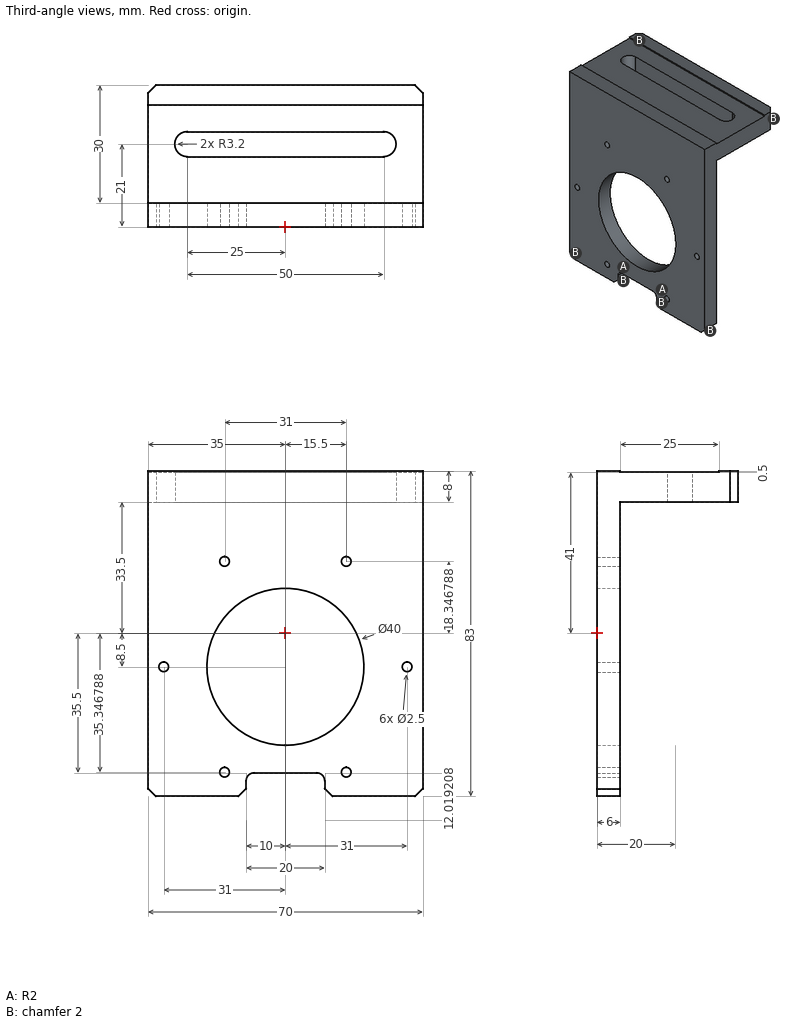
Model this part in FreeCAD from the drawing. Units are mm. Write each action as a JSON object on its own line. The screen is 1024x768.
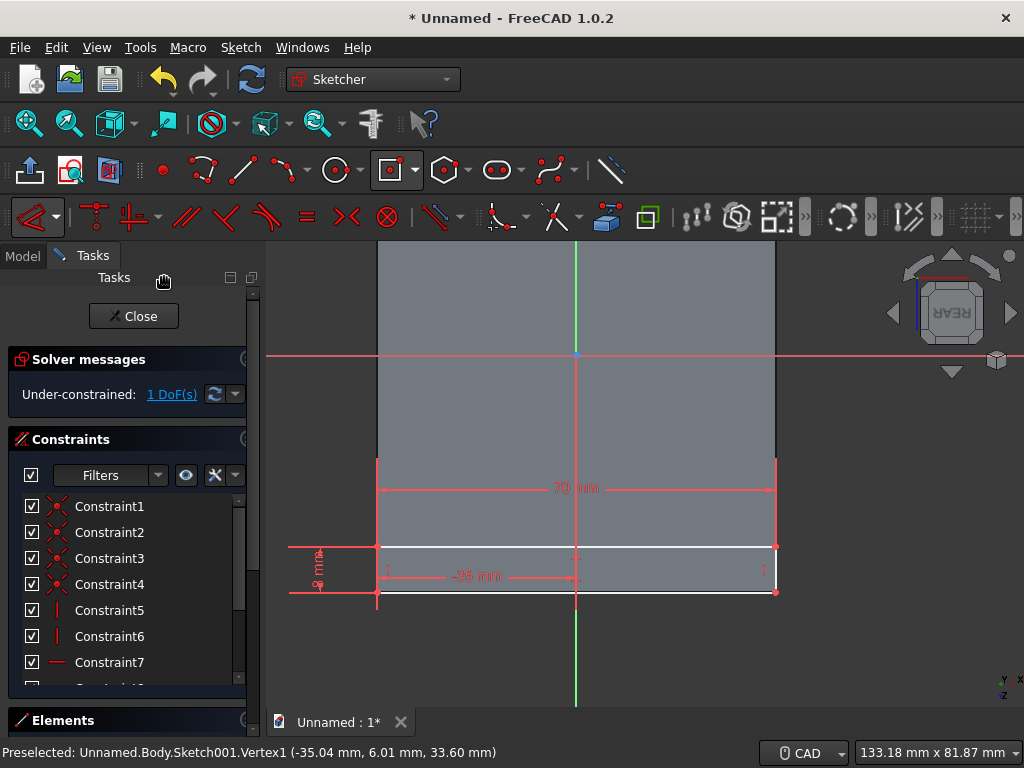
{"action": "left_click", "coordinate": [377, 547]}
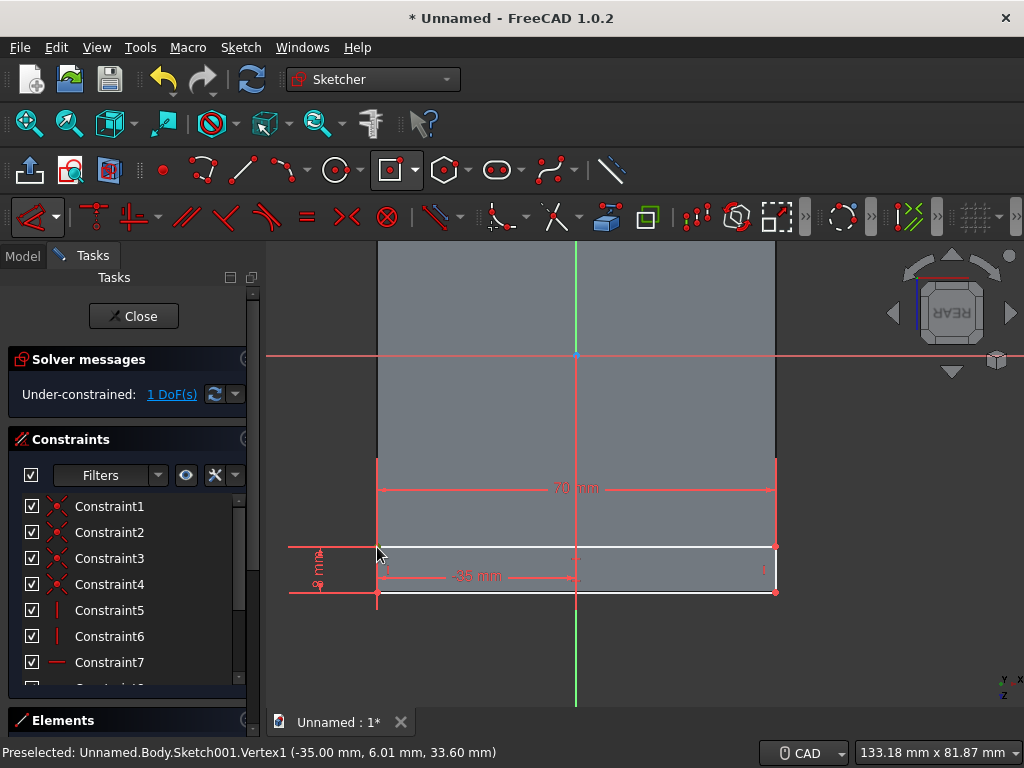
{"action": "left_click", "coordinate": [58, 218]}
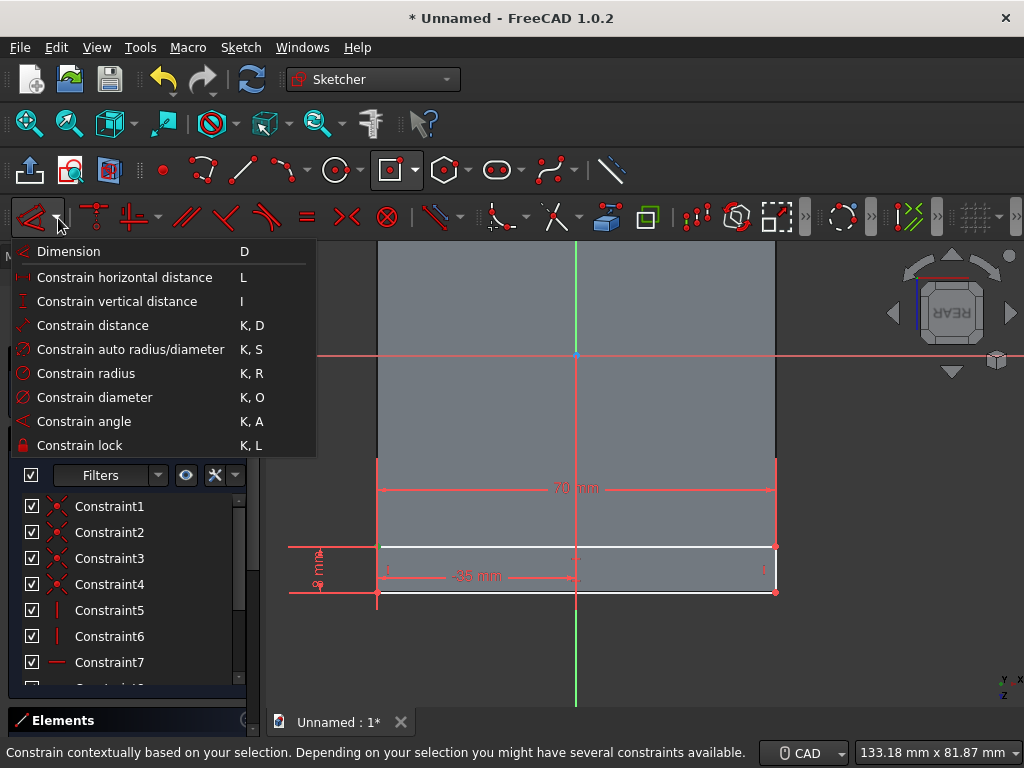
{"action": "left_click", "coordinate": [164, 301]}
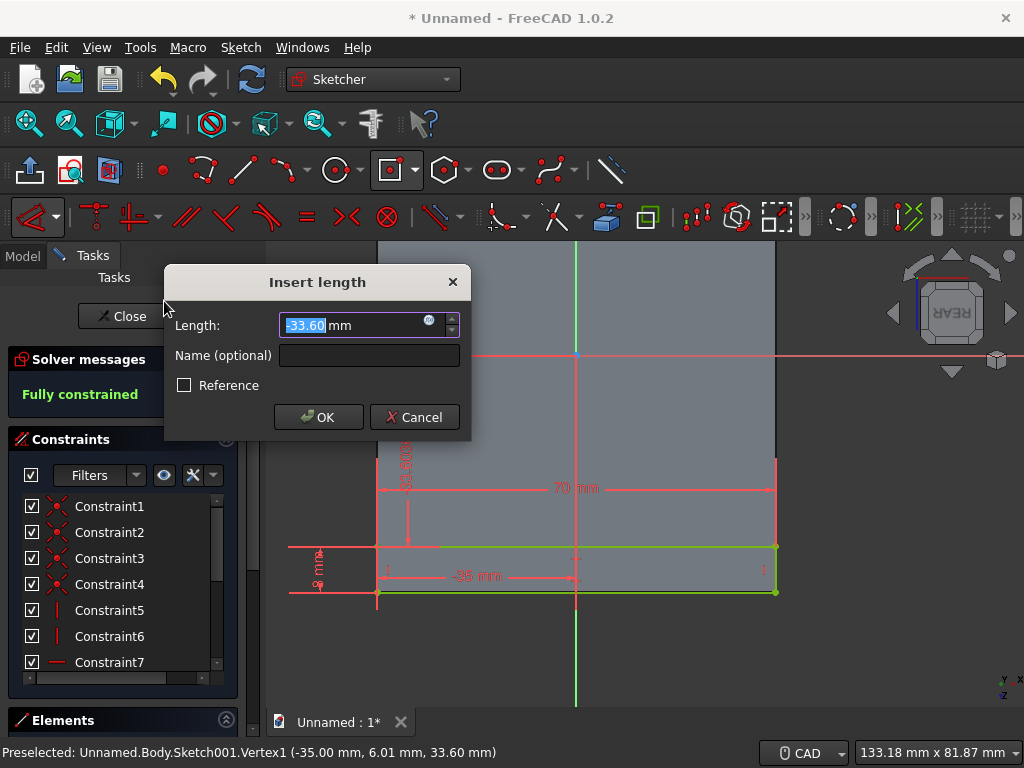
{"action": "type", "text": "-33.5"}
{"action": "key", "text": "Return"}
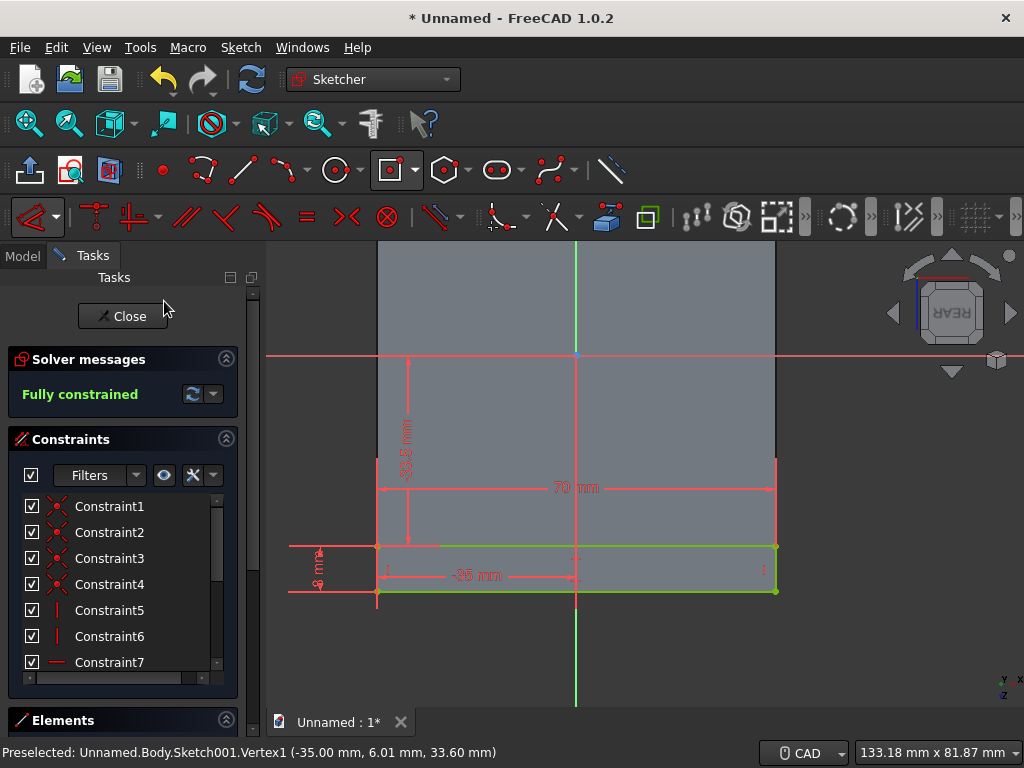
{"action": "left_click", "coordinate": [123, 316]}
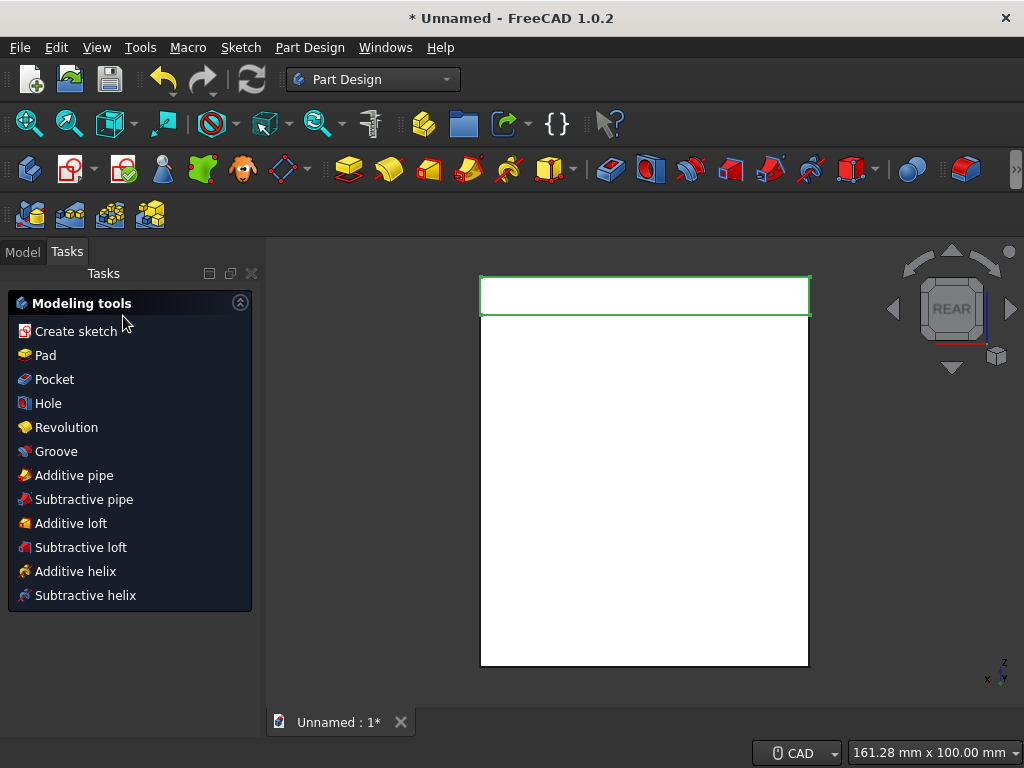
{"action": "left_click", "coordinate": [350, 170]}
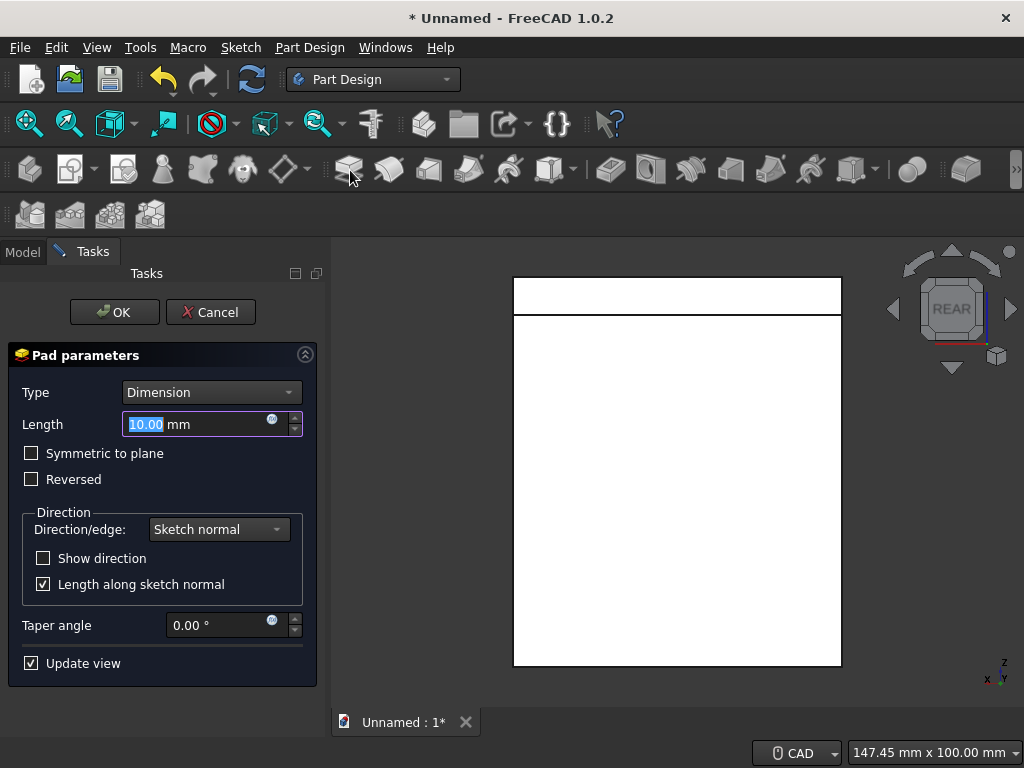
{"action": "type", "text": "30"}
{"action": "key", "text": "Tab"}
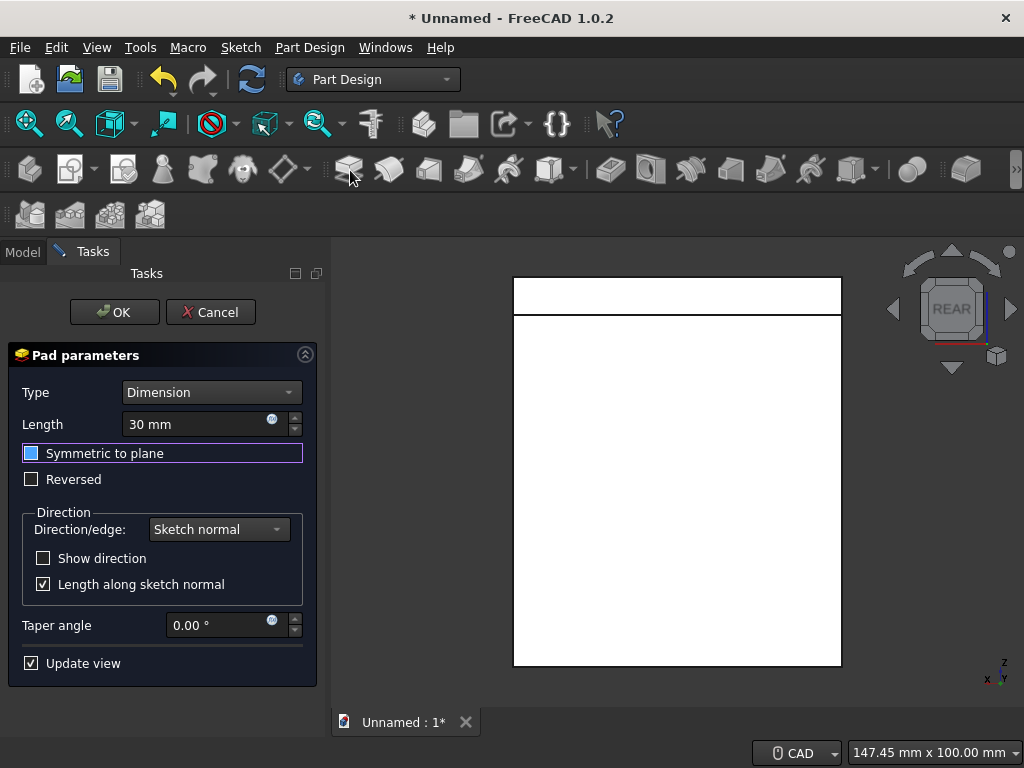
{"action": "left_click", "coordinate": [115, 312]}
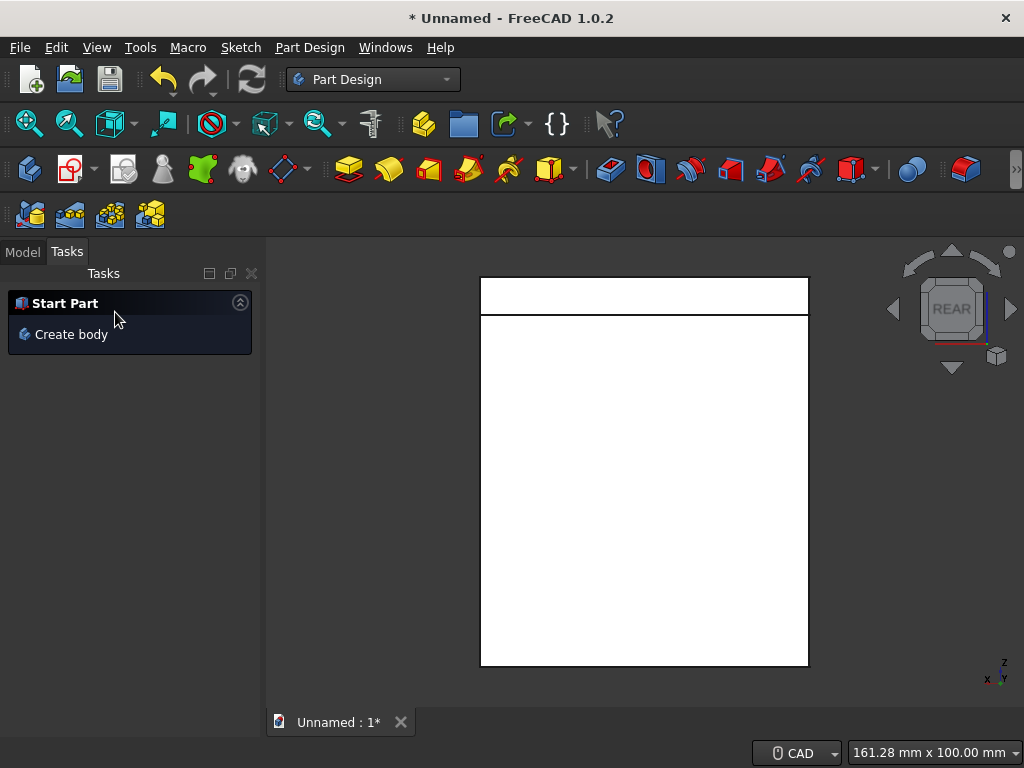
{"action": "left_click", "coordinate": [70, 170]}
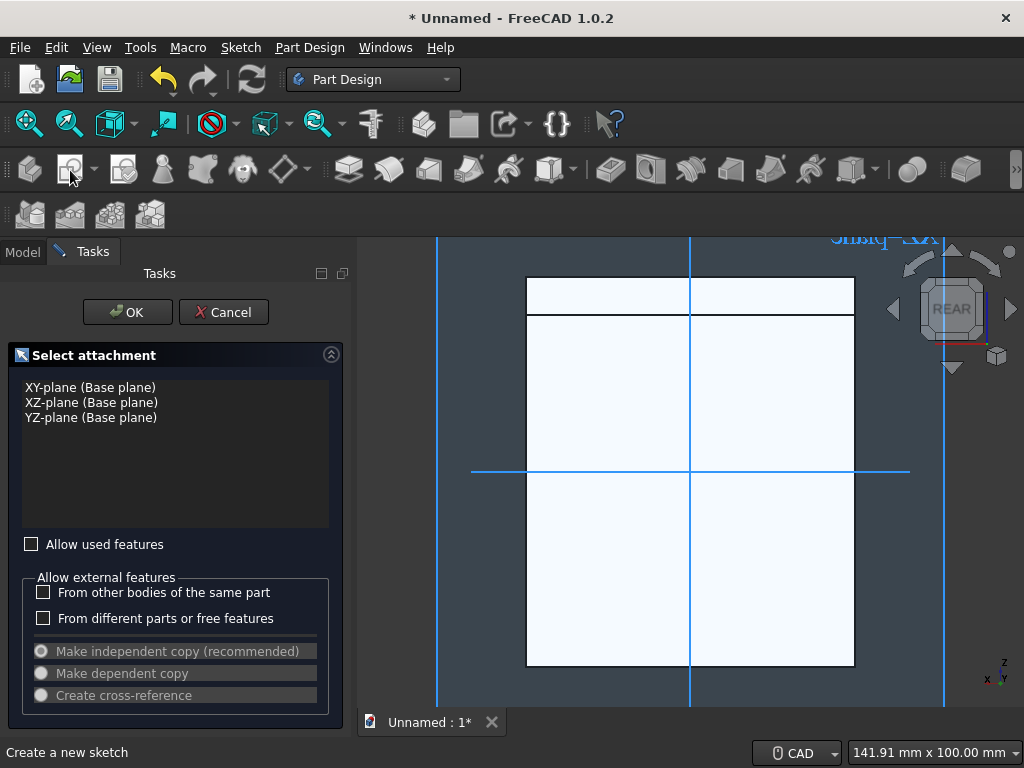
{"action": "left_click", "coordinate": [82, 402]}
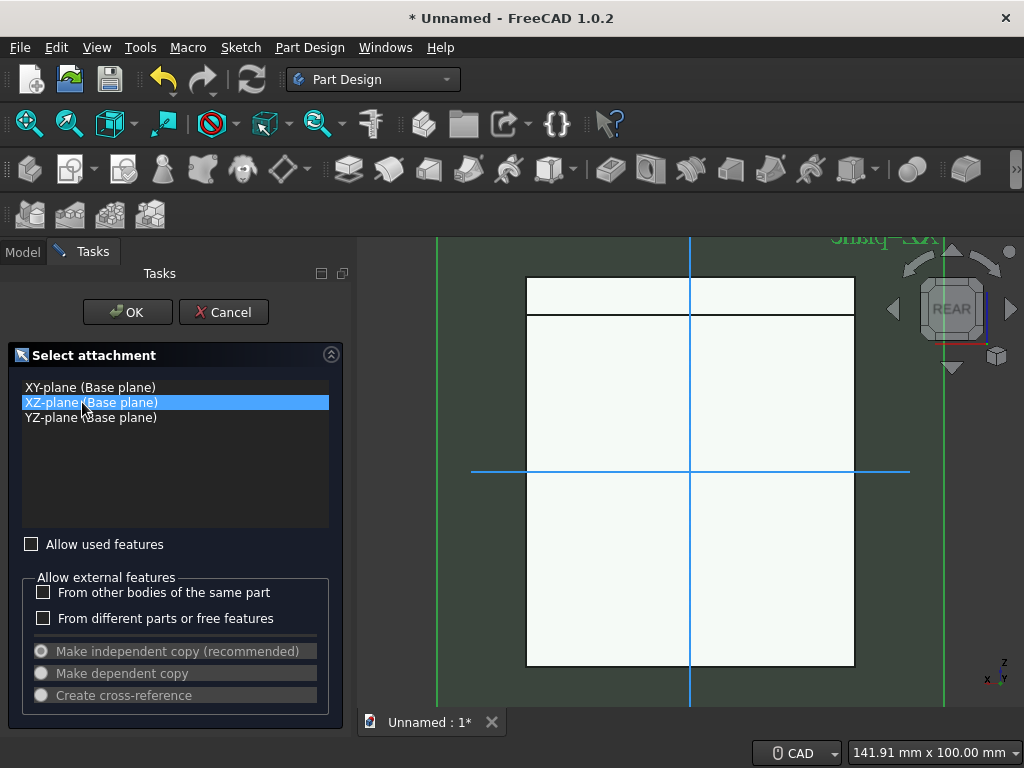
{"action": "left_click", "coordinate": [128, 312]}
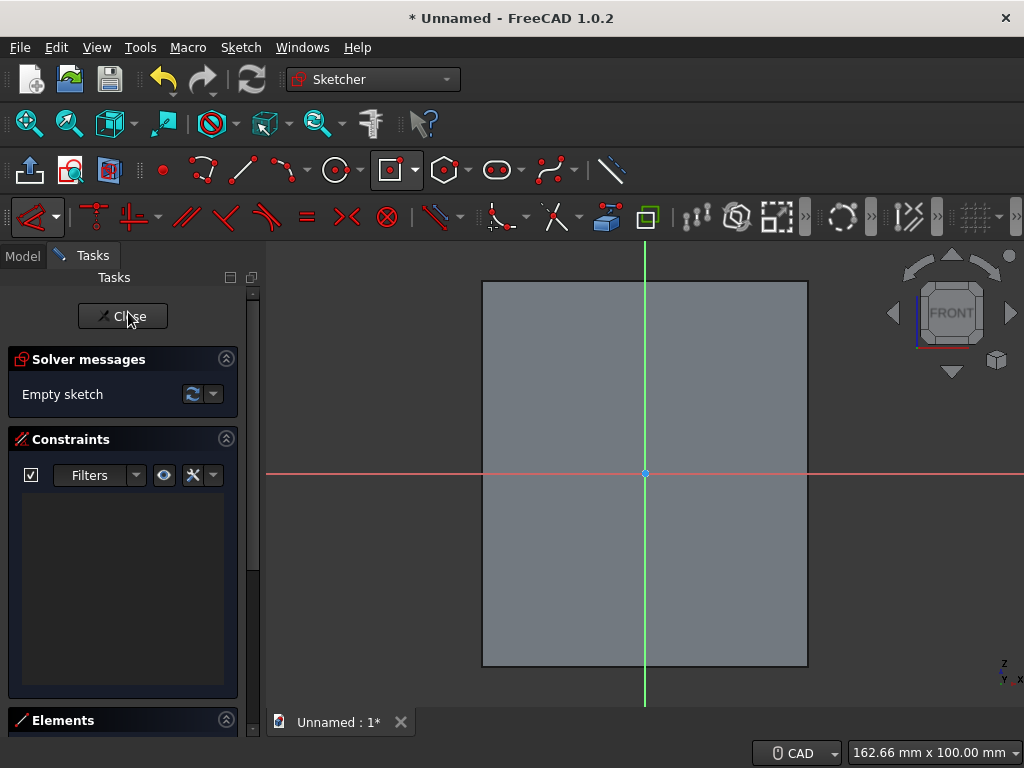
{"action": "scroll", "coordinate": [784, 594], "scroll_direction": "up", "scroll_amount": 2}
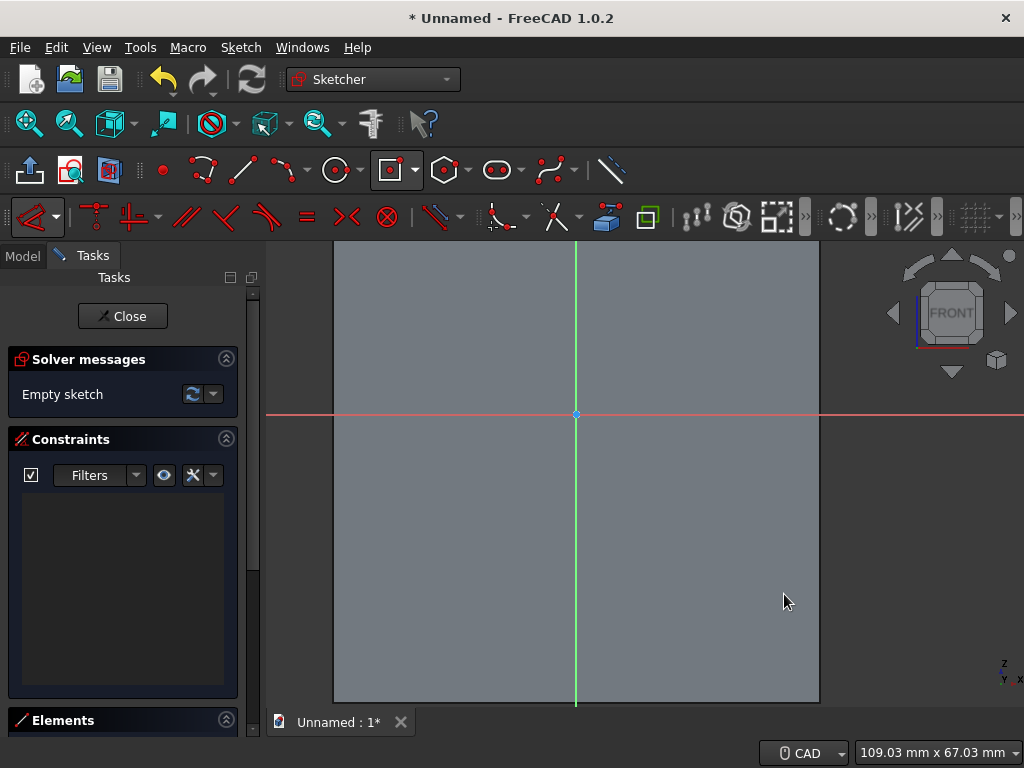
{"action": "left_click", "coordinate": [336, 170]}